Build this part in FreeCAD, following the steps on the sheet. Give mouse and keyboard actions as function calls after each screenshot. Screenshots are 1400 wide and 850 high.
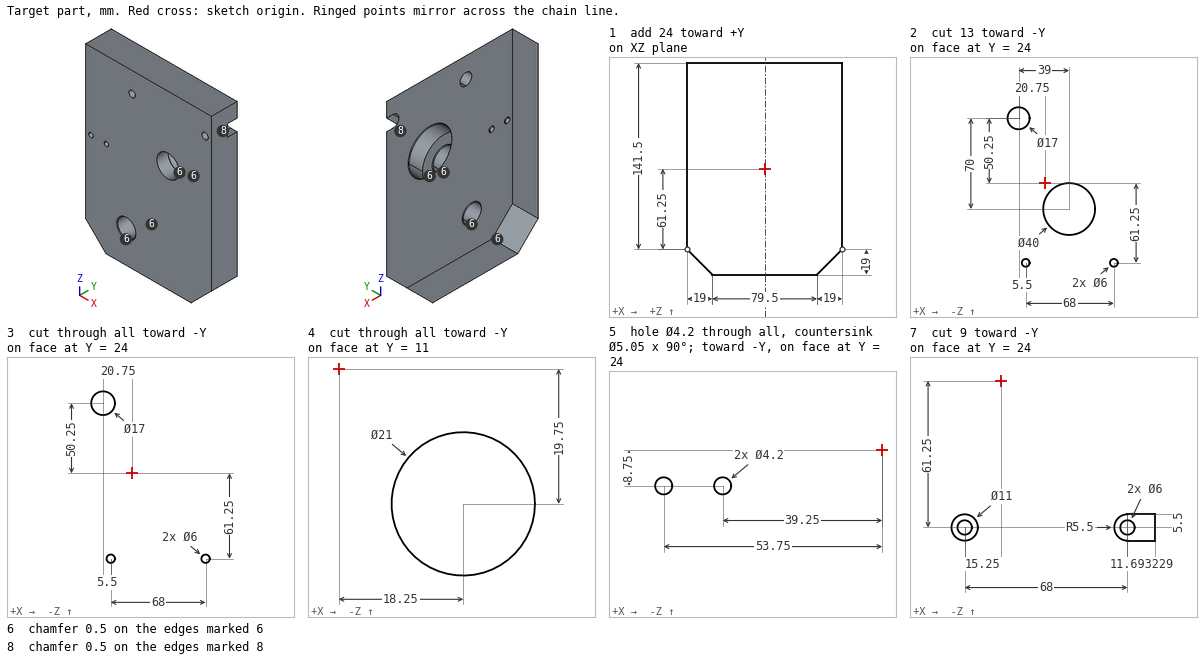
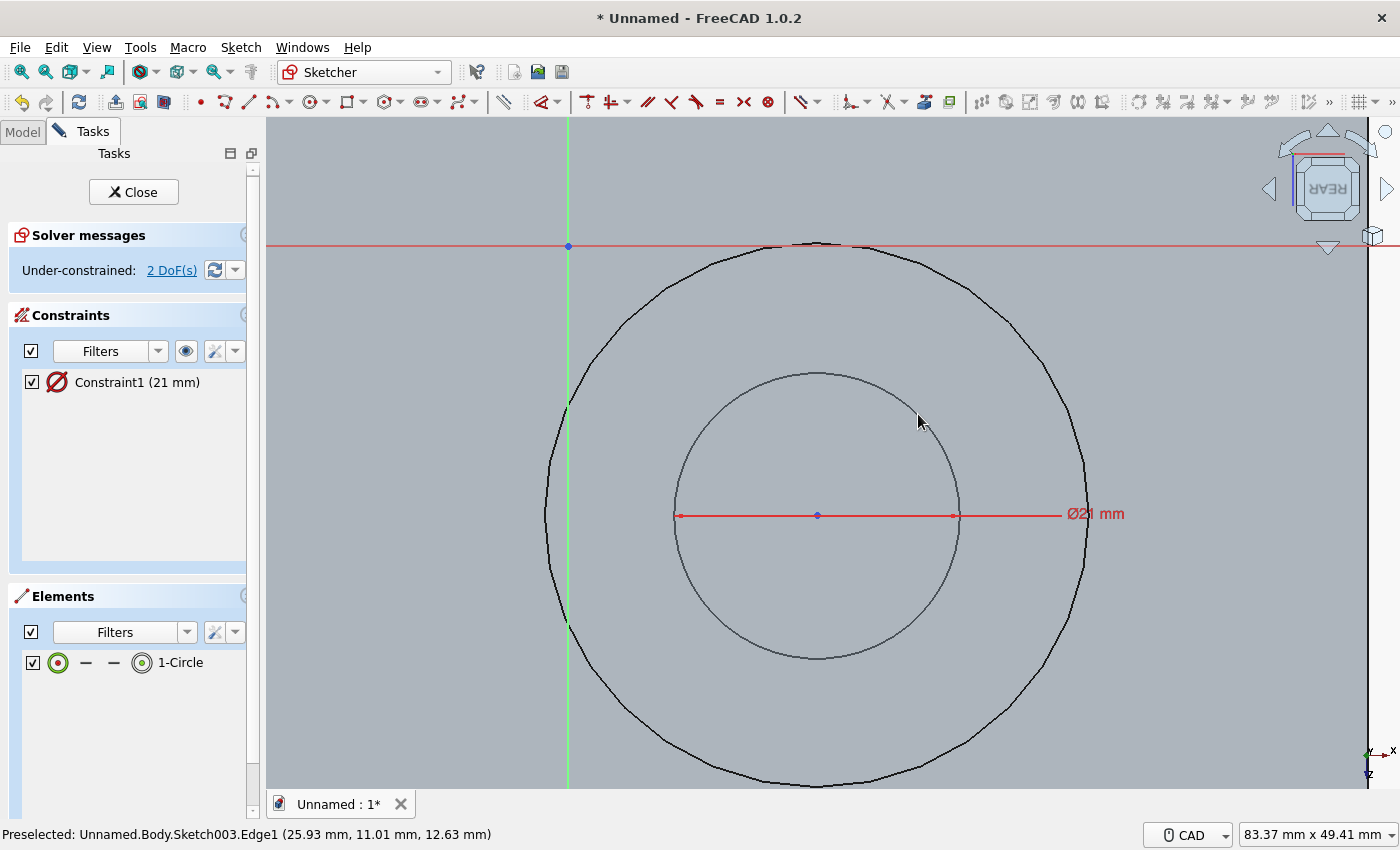
click(542, 102)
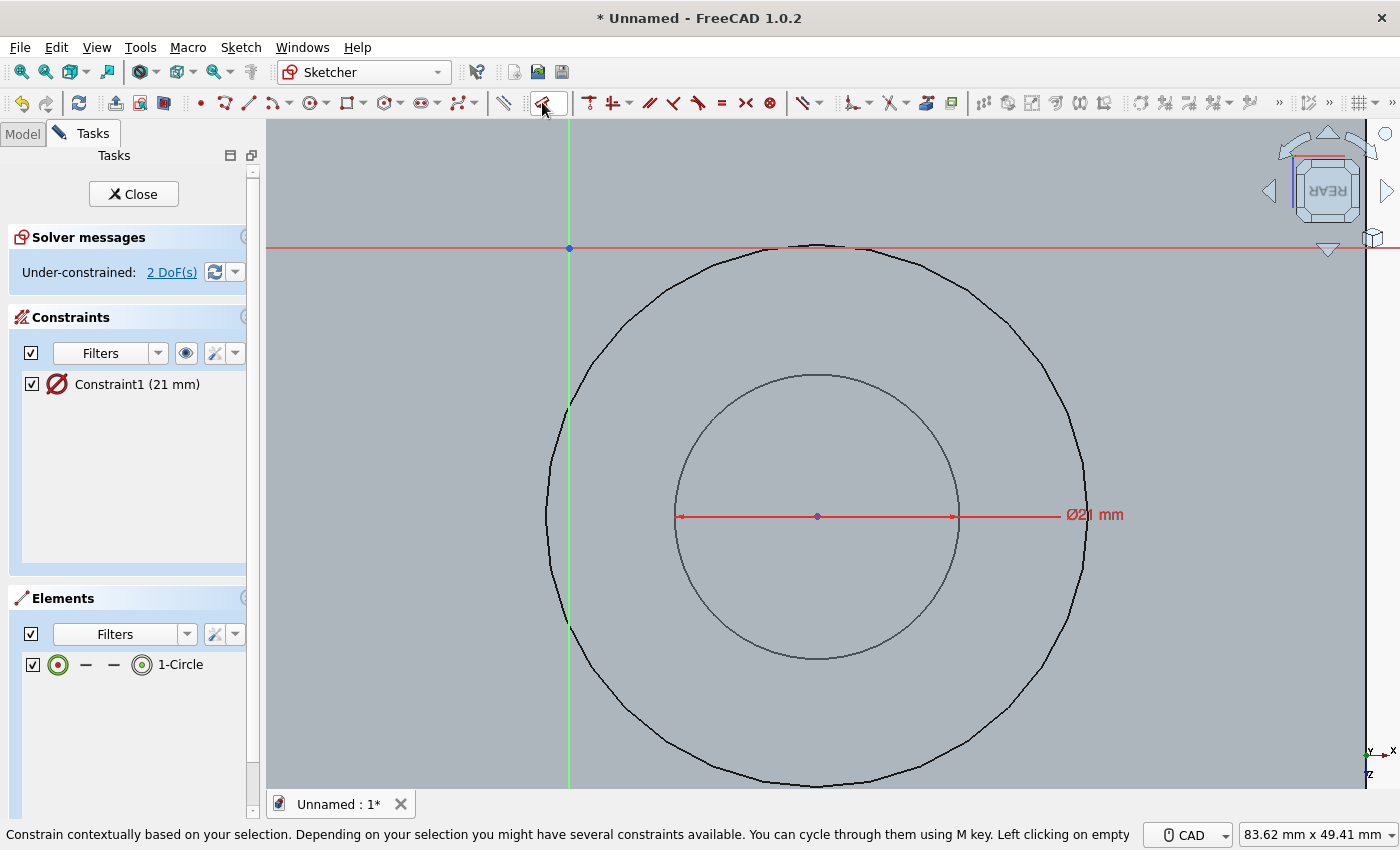
click(817, 517)
click(693, 214)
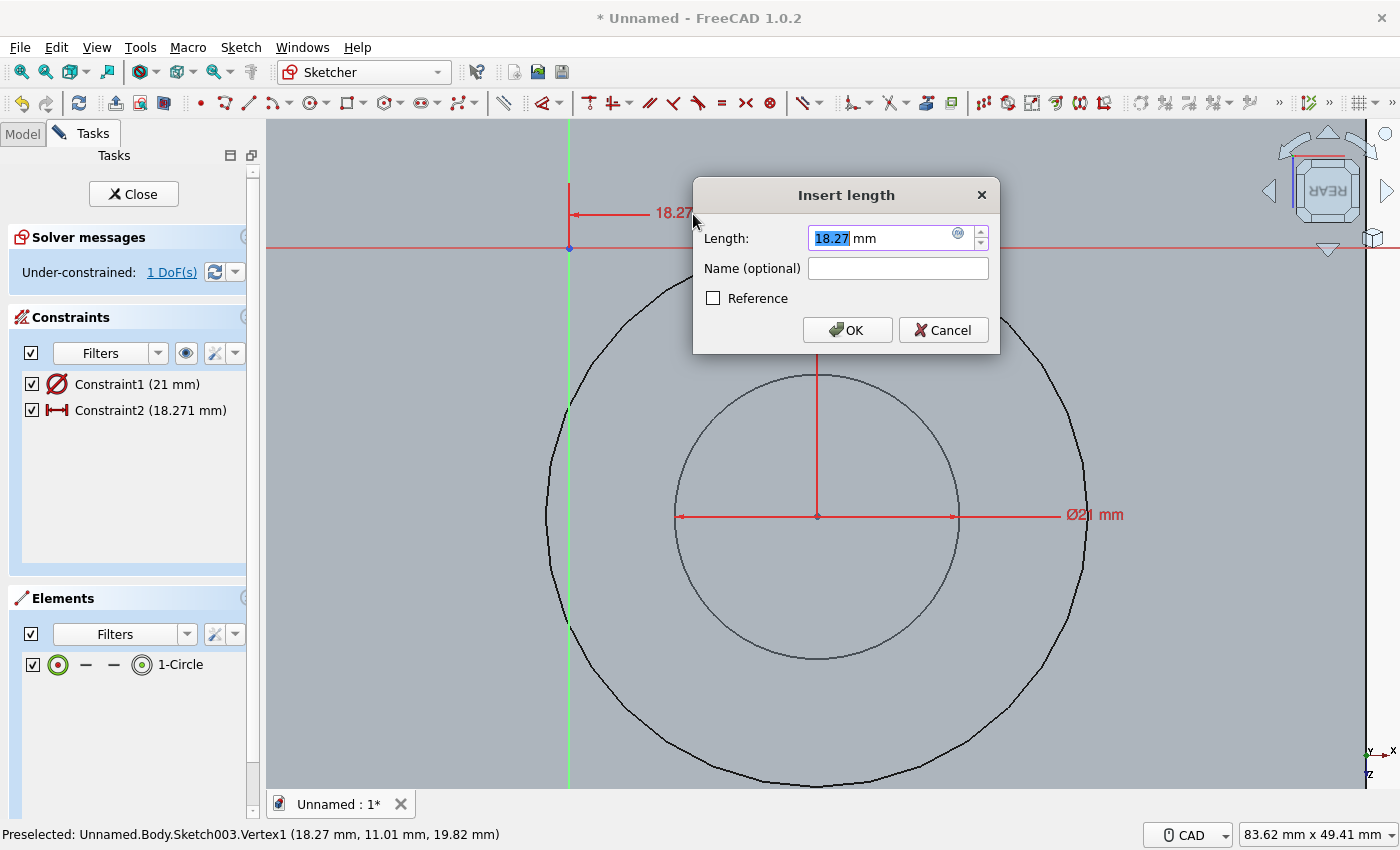
text(18.25)
key(Return)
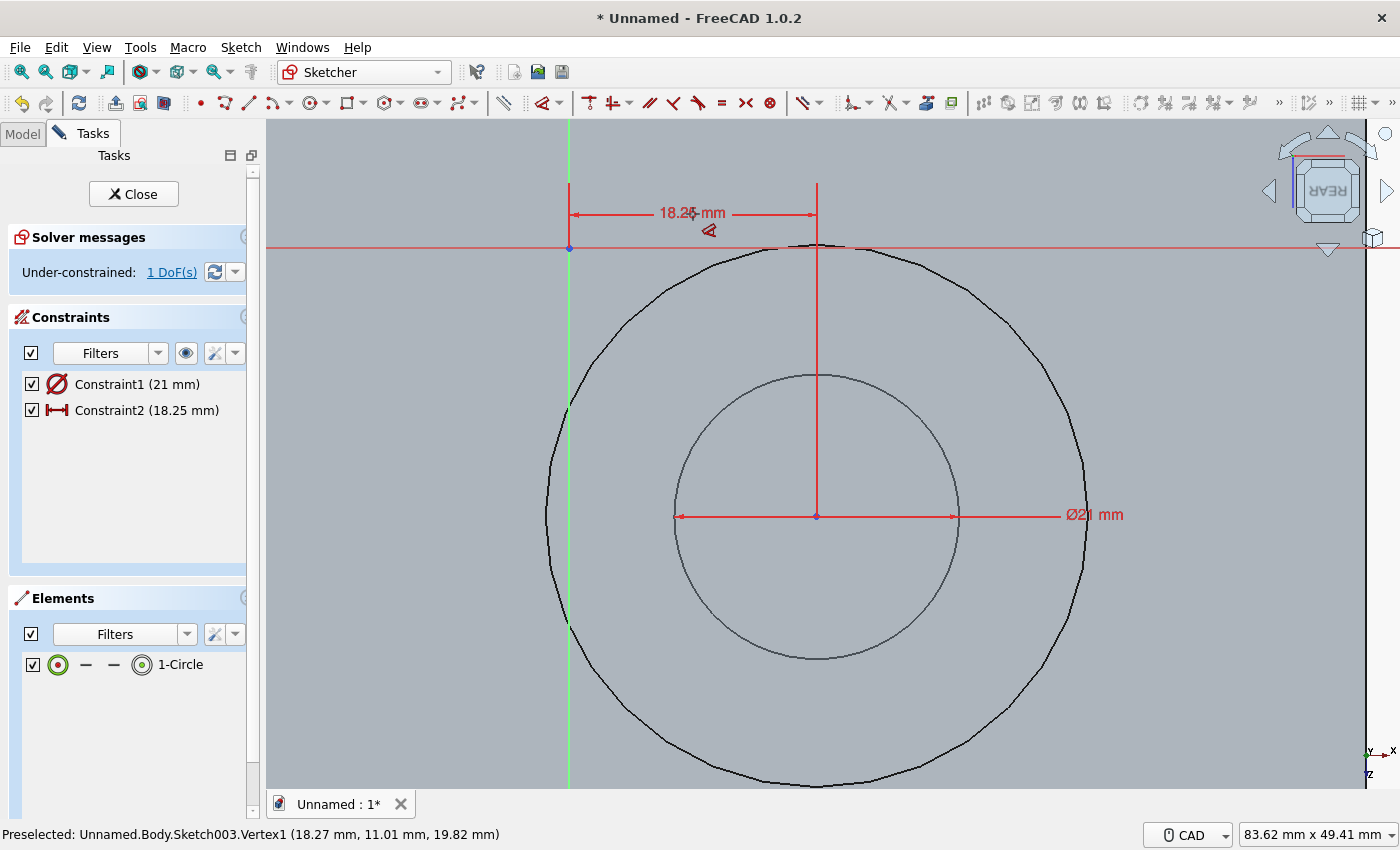
click(817, 517)
click(535, 382)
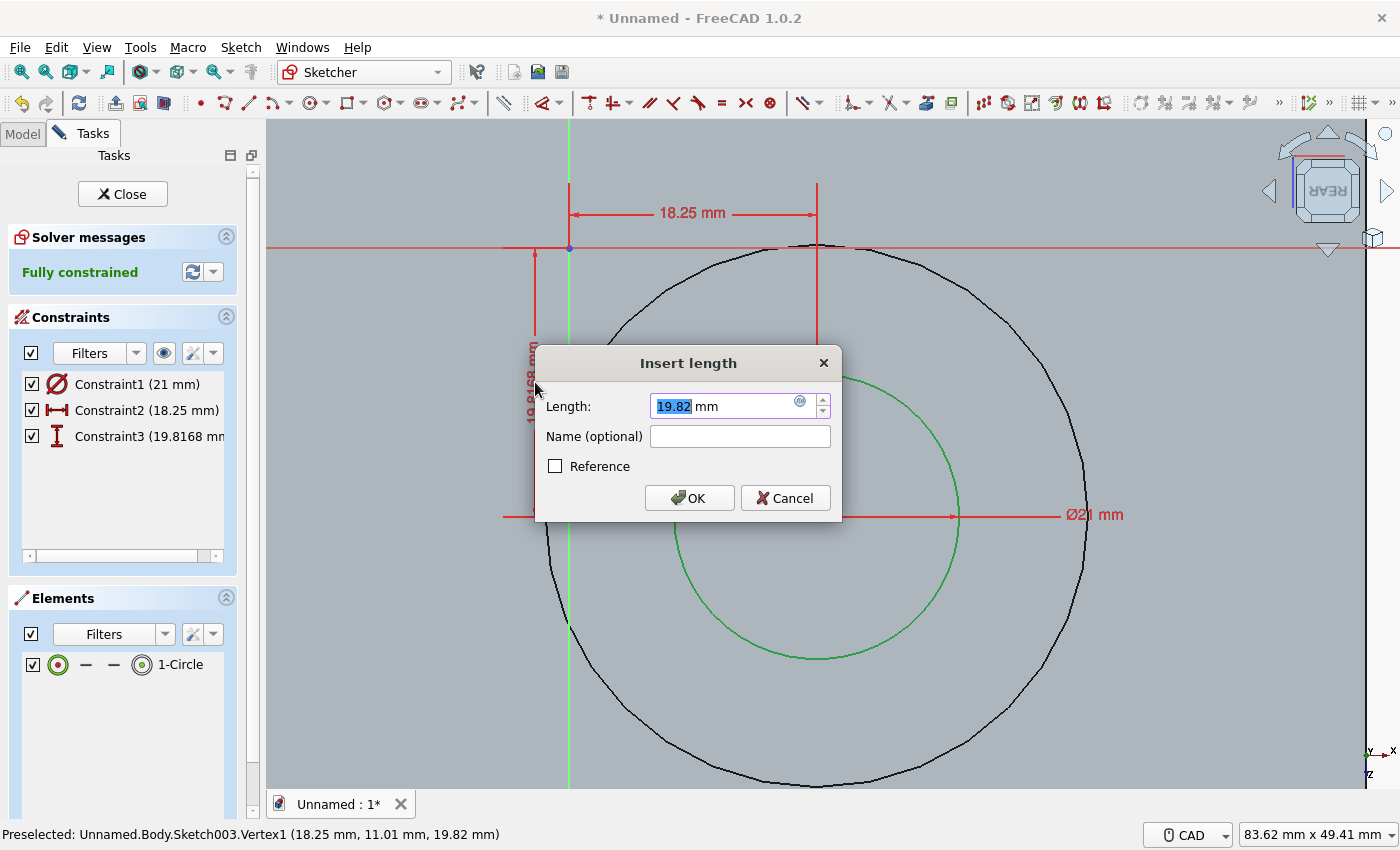
text(19.75)
key(Return)
key(Escape)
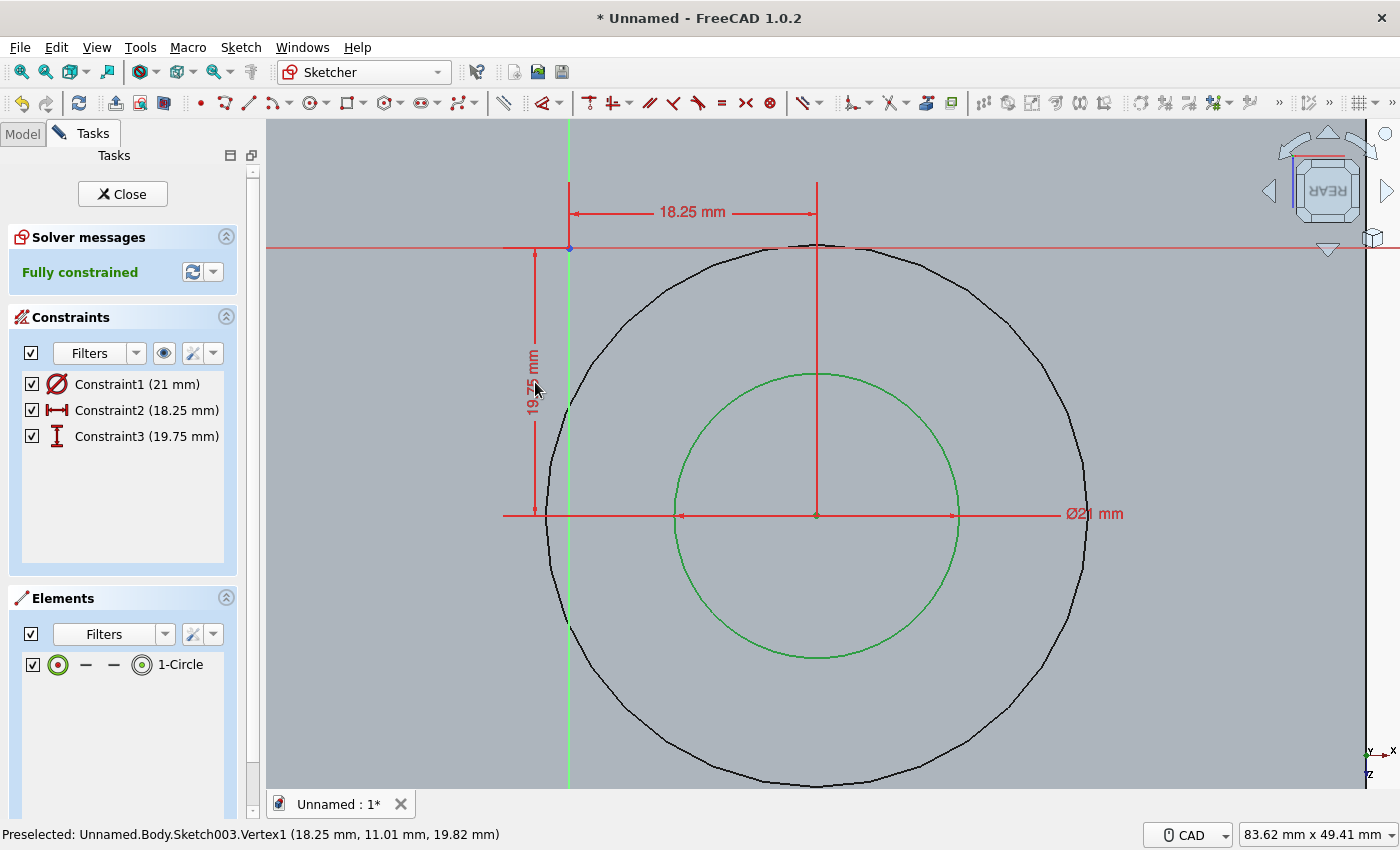
click(123, 194)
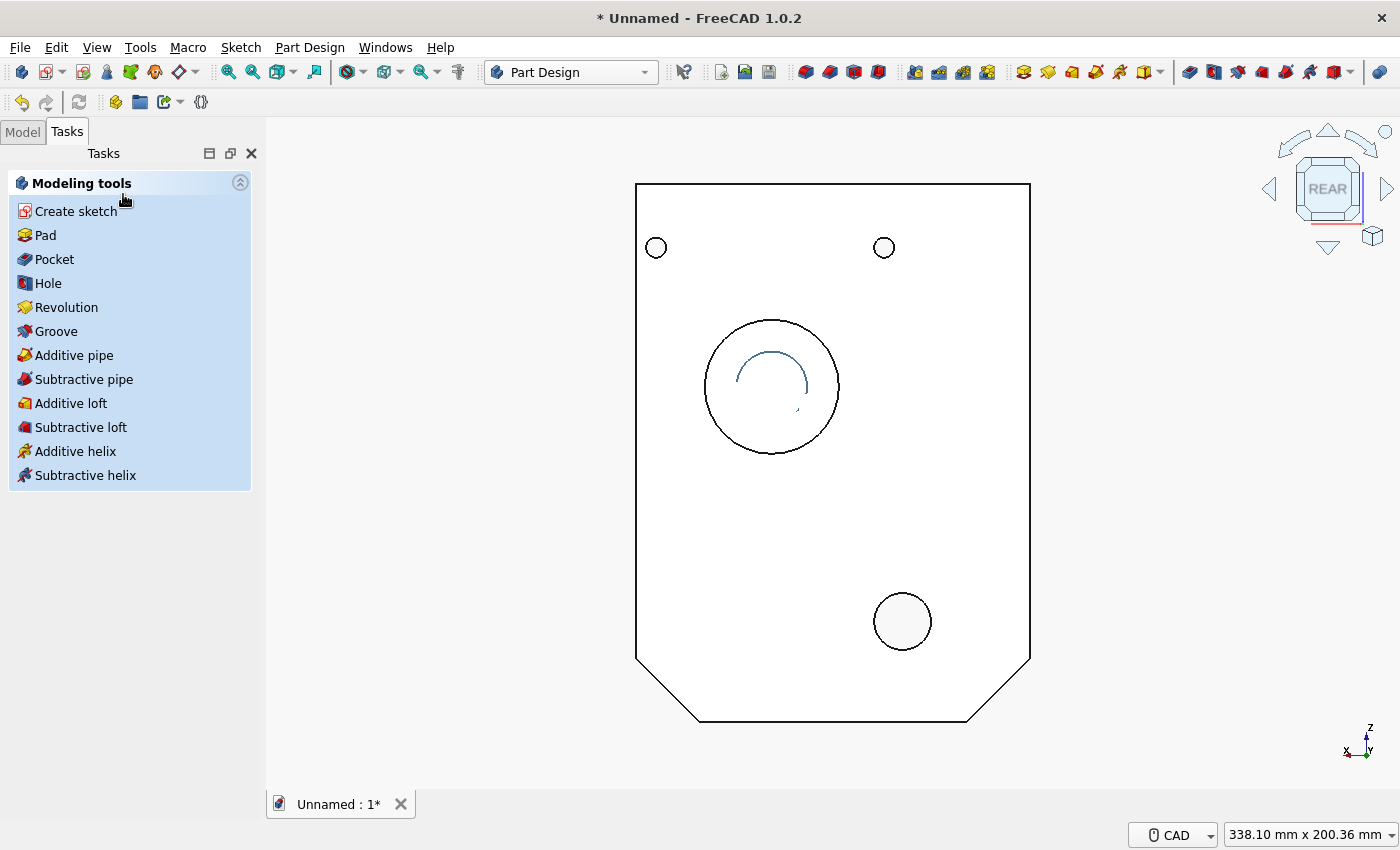
click(1190, 72)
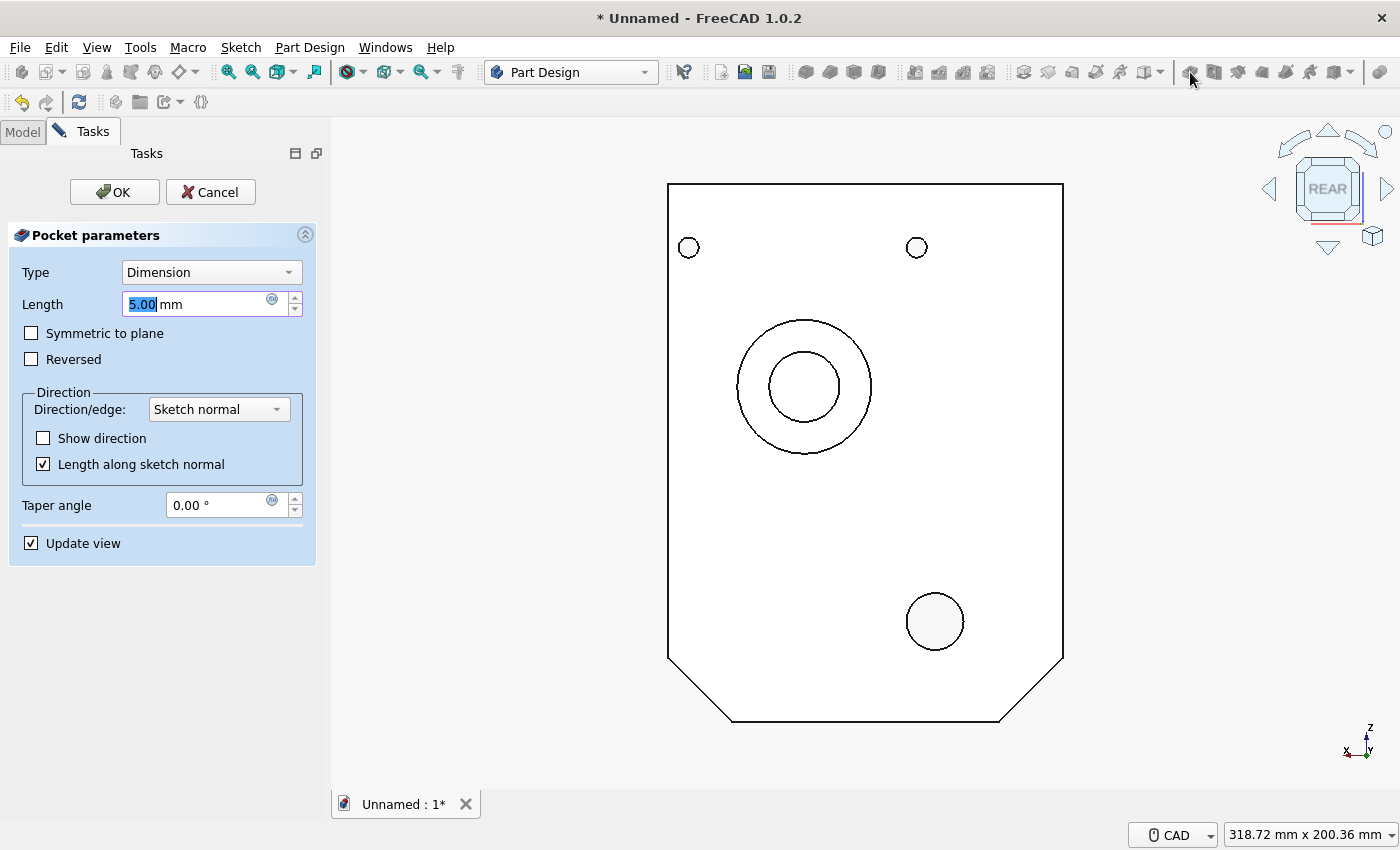
click(212, 272)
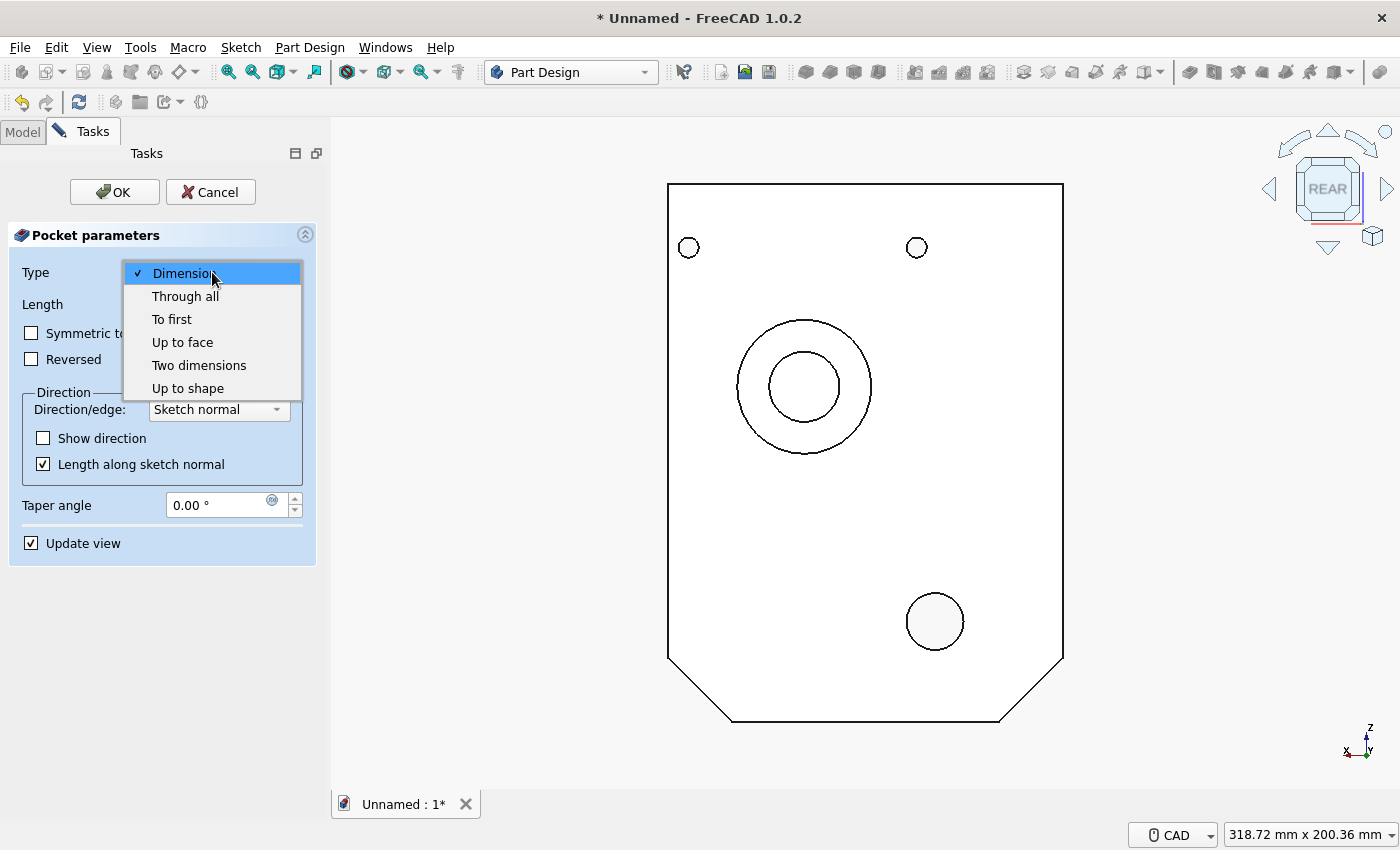
click(212, 296)